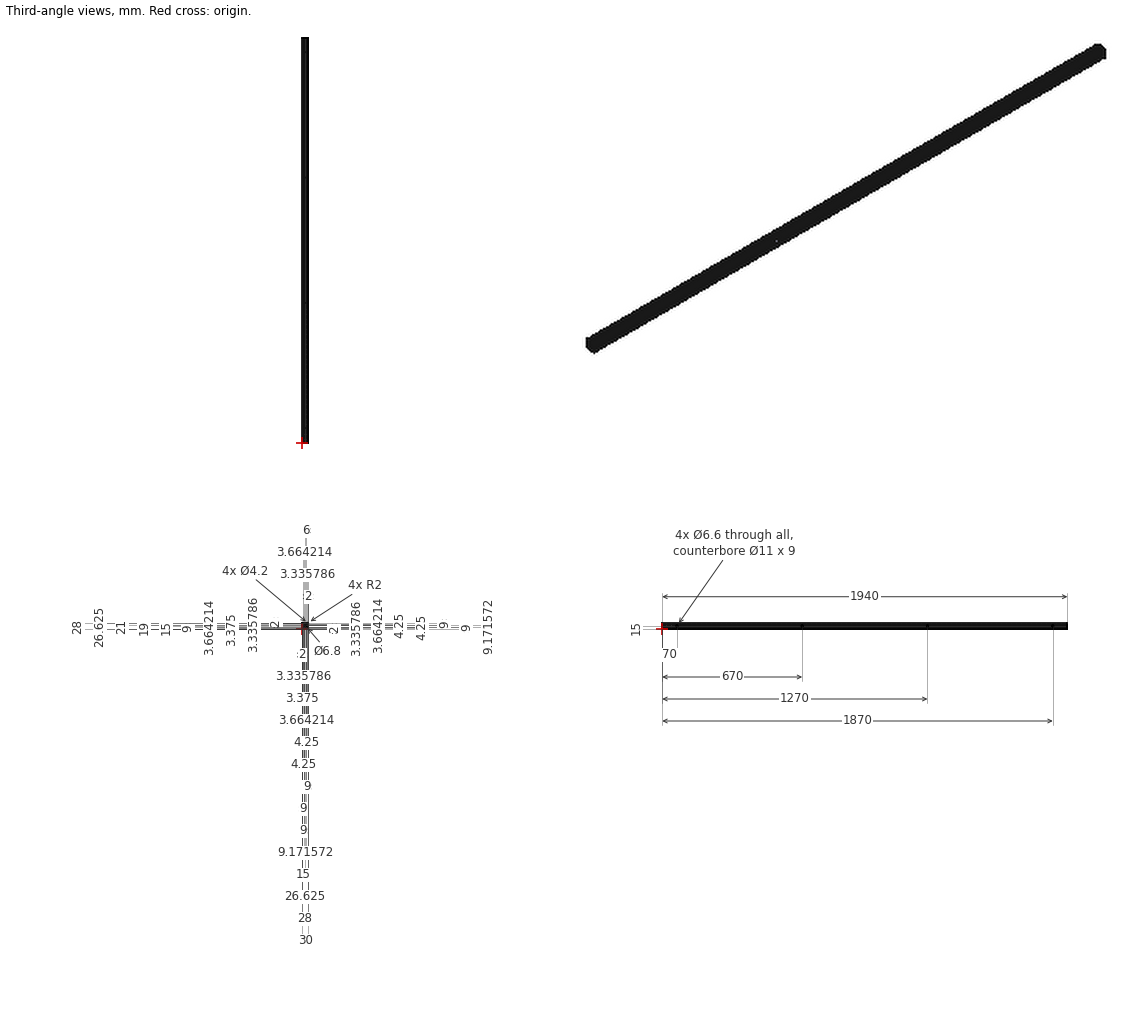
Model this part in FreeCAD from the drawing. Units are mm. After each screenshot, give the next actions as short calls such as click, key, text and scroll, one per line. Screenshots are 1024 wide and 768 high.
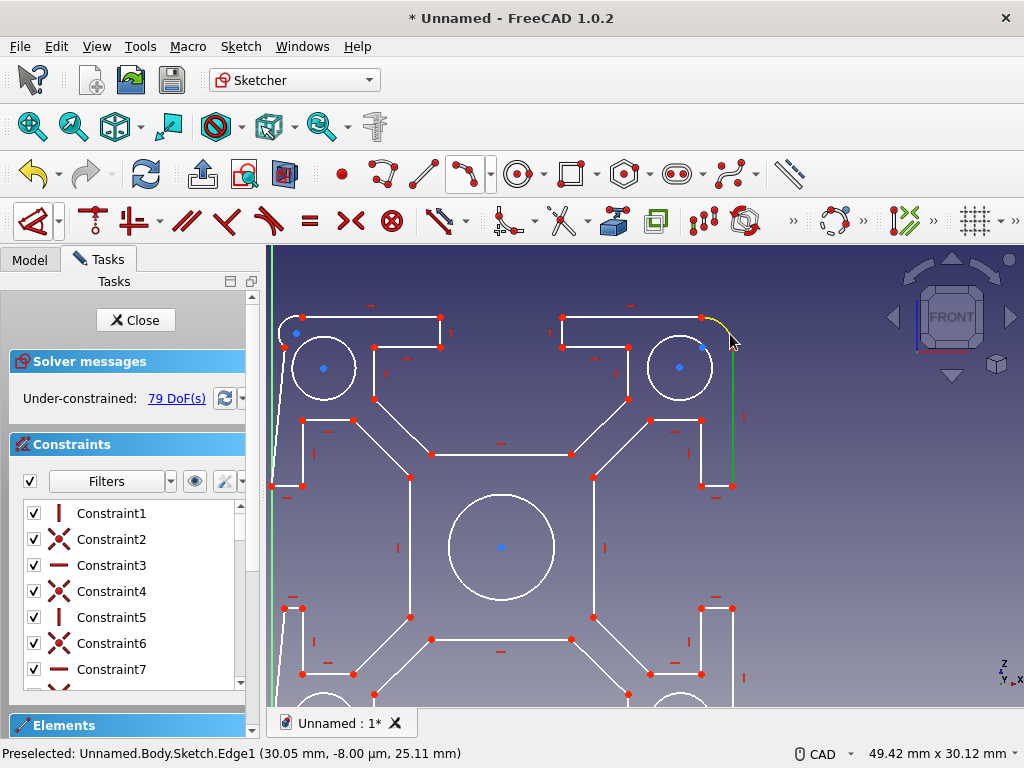
click(729, 333)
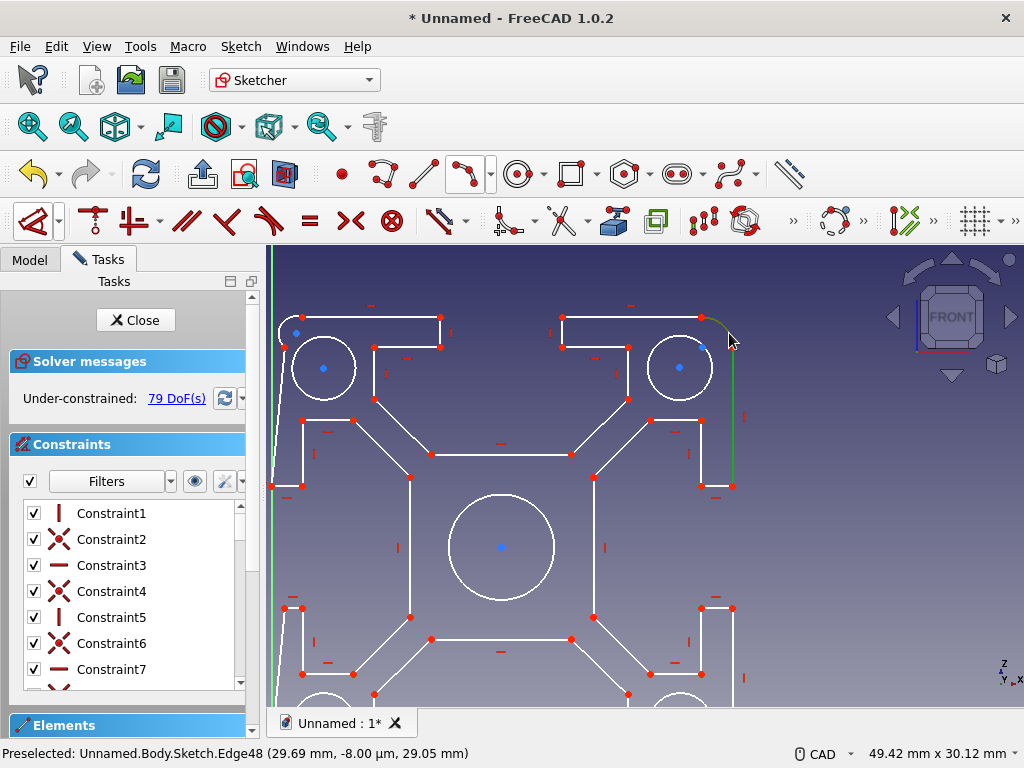
click(269, 222)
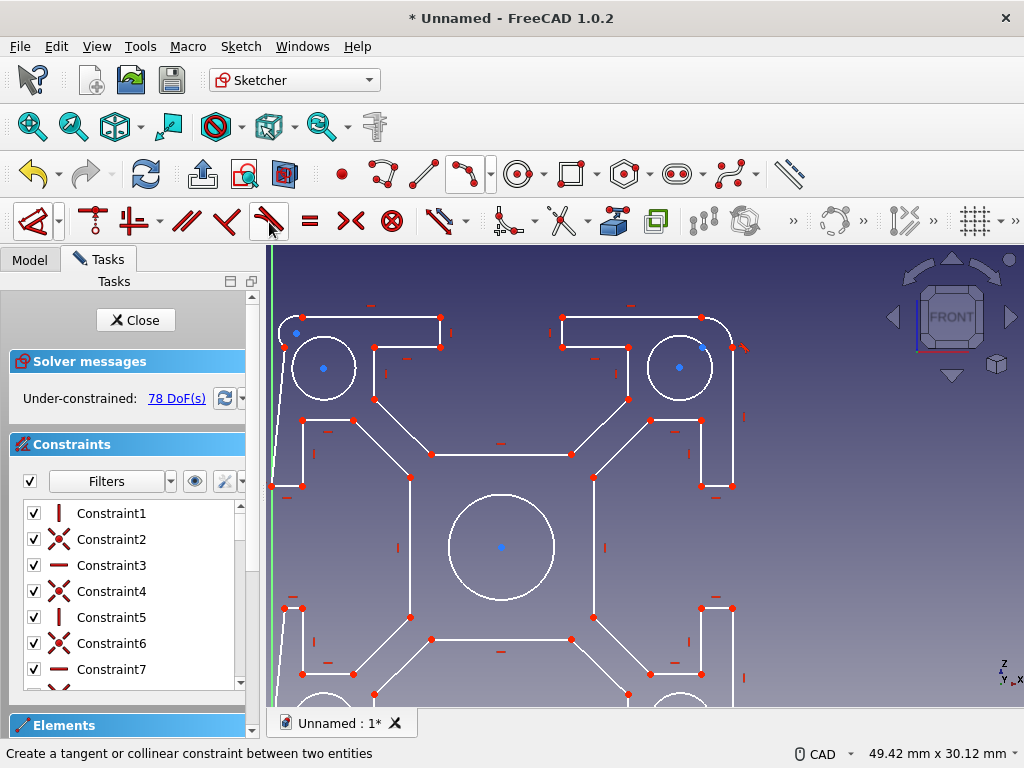
click(733, 650)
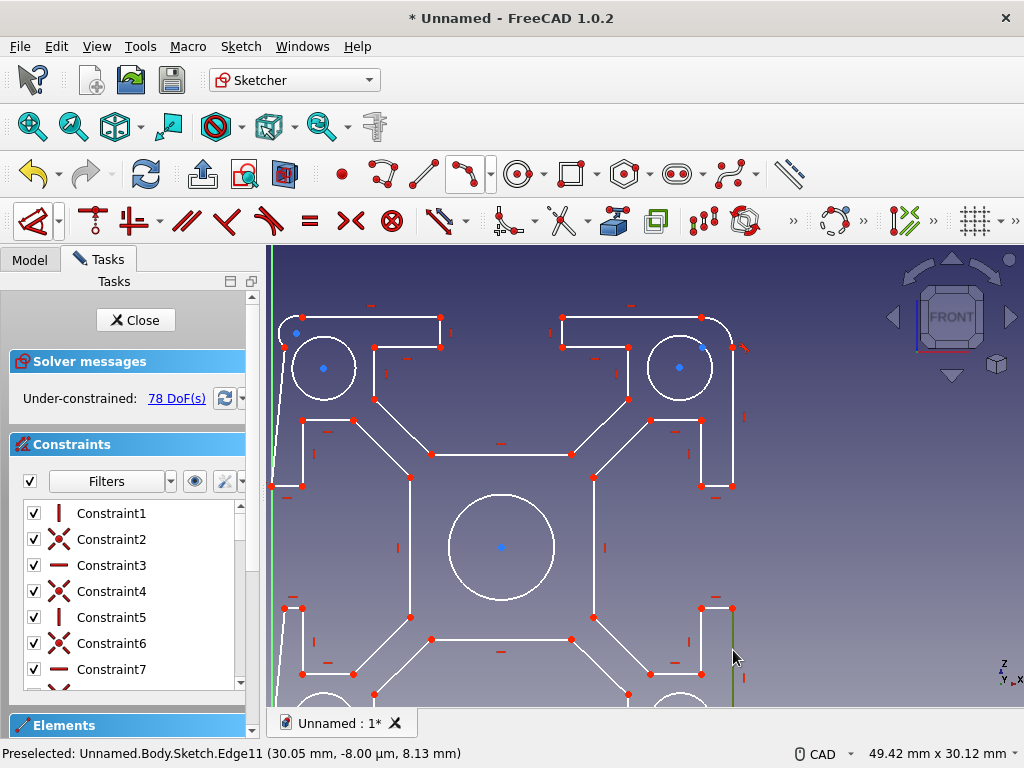
scroll(729, 334, down, 2)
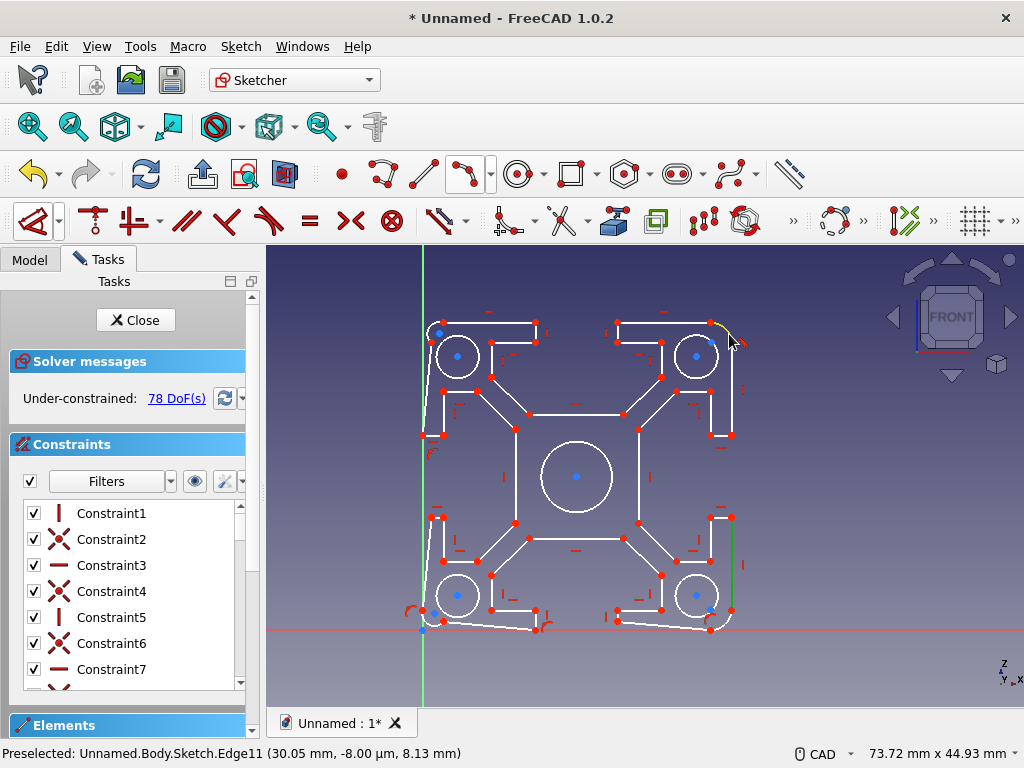
scroll(720, 628, up, 2)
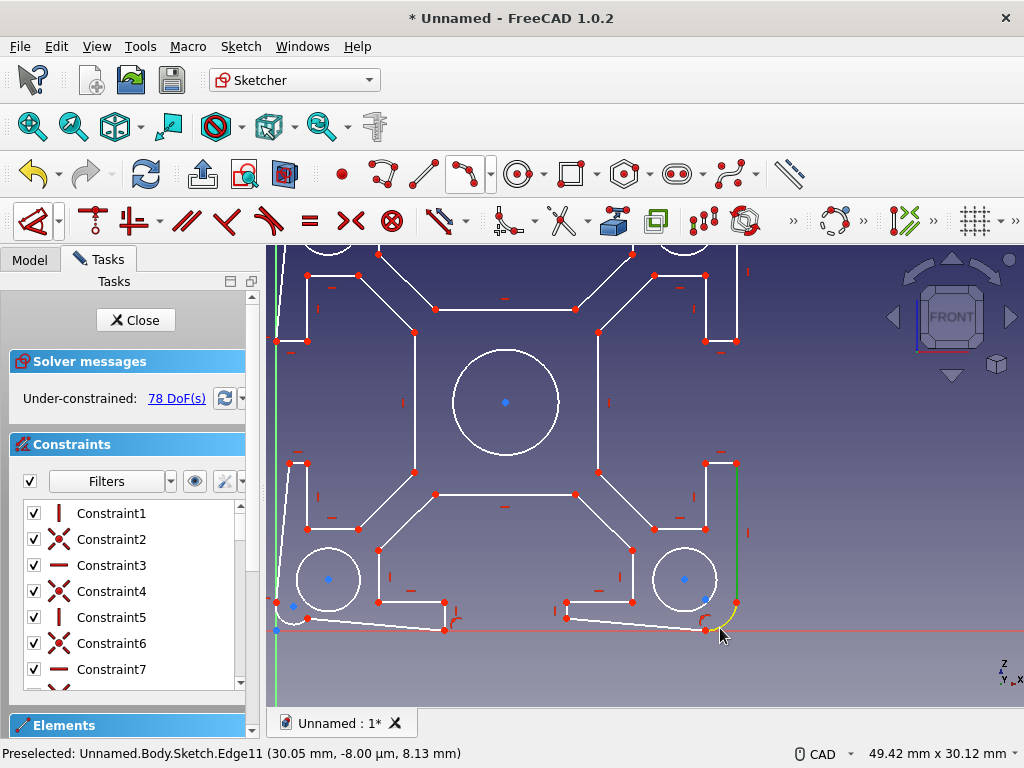
click(719, 628)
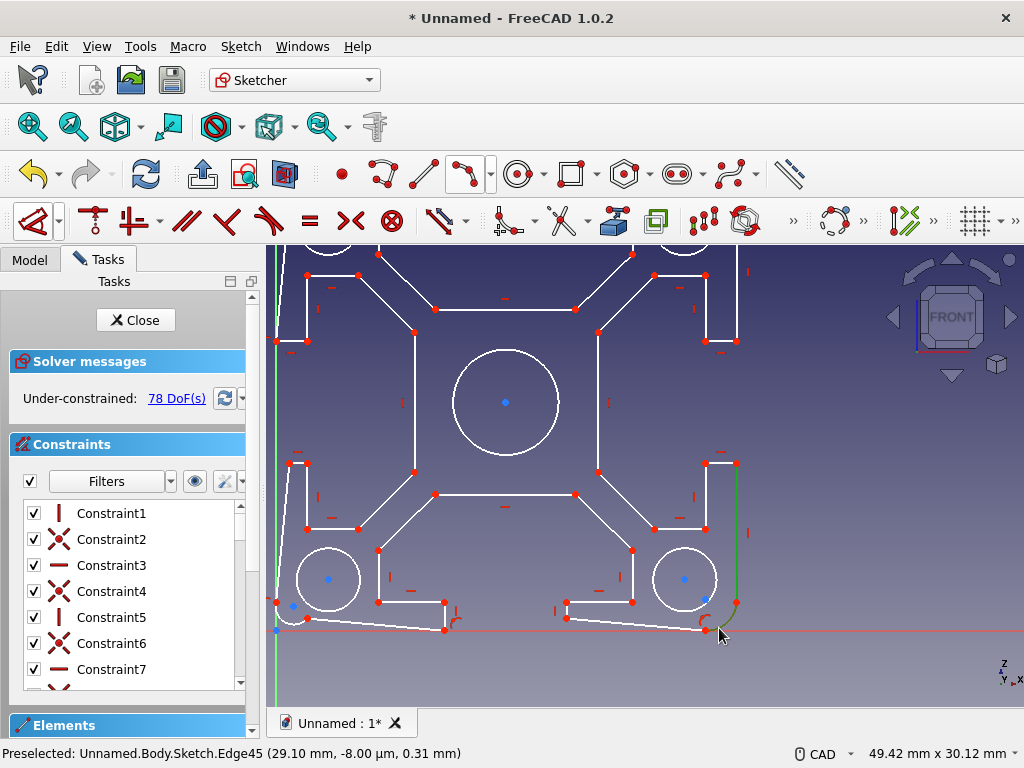
key(t)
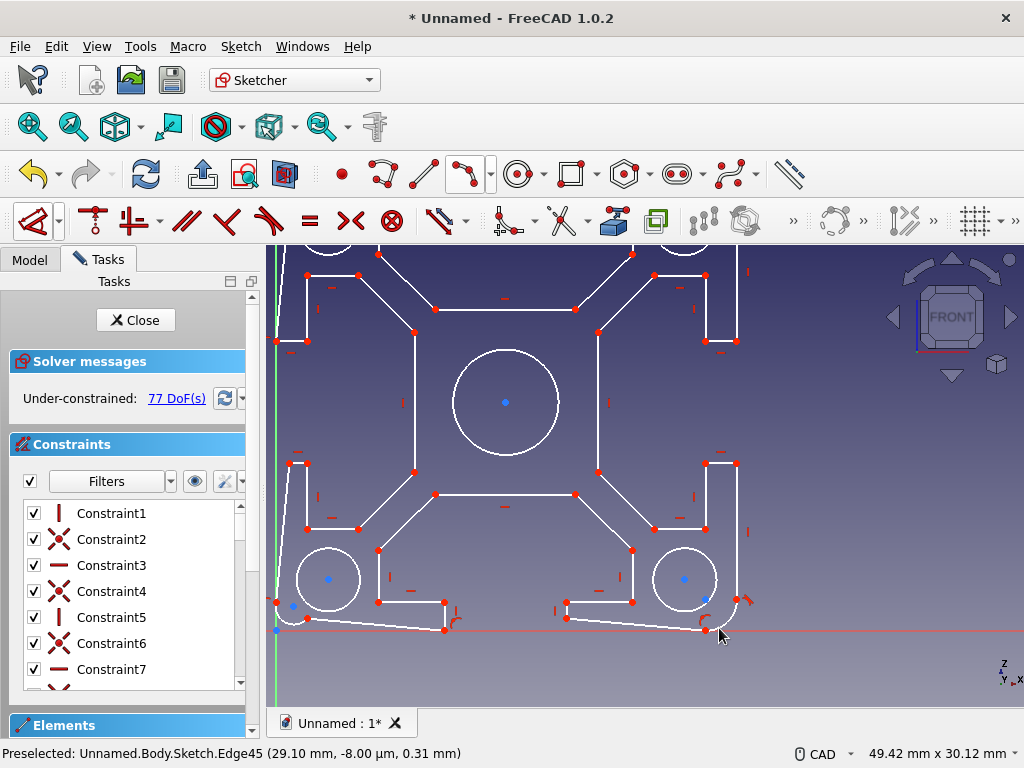
click(664, 627)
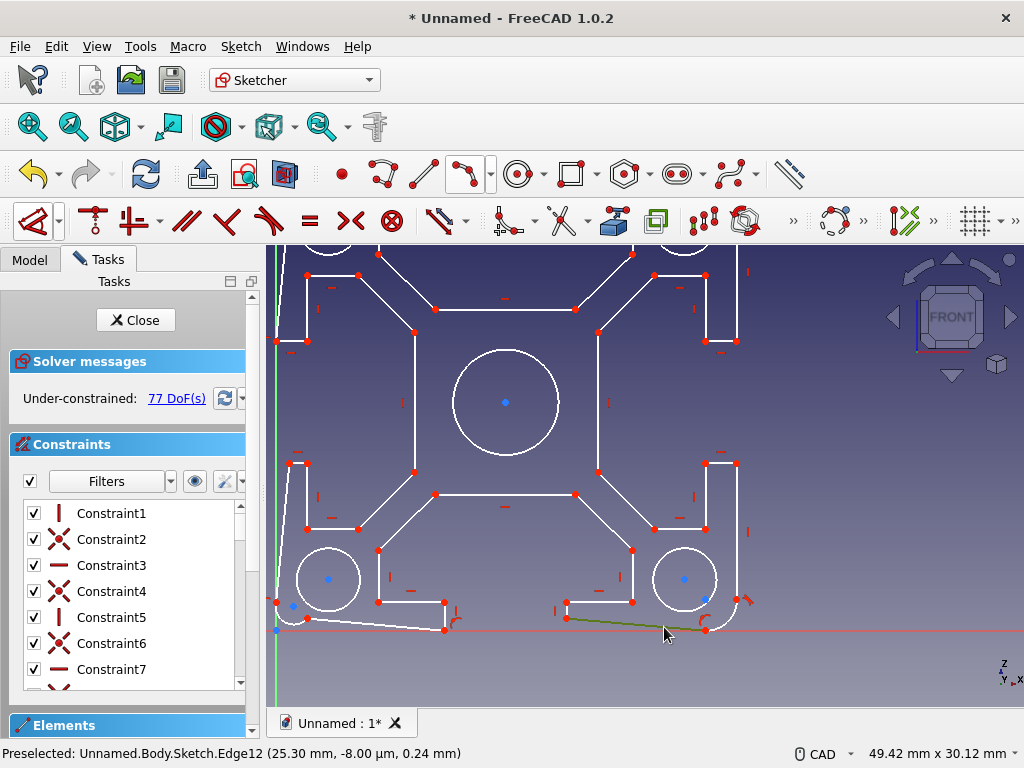
click(720, 627)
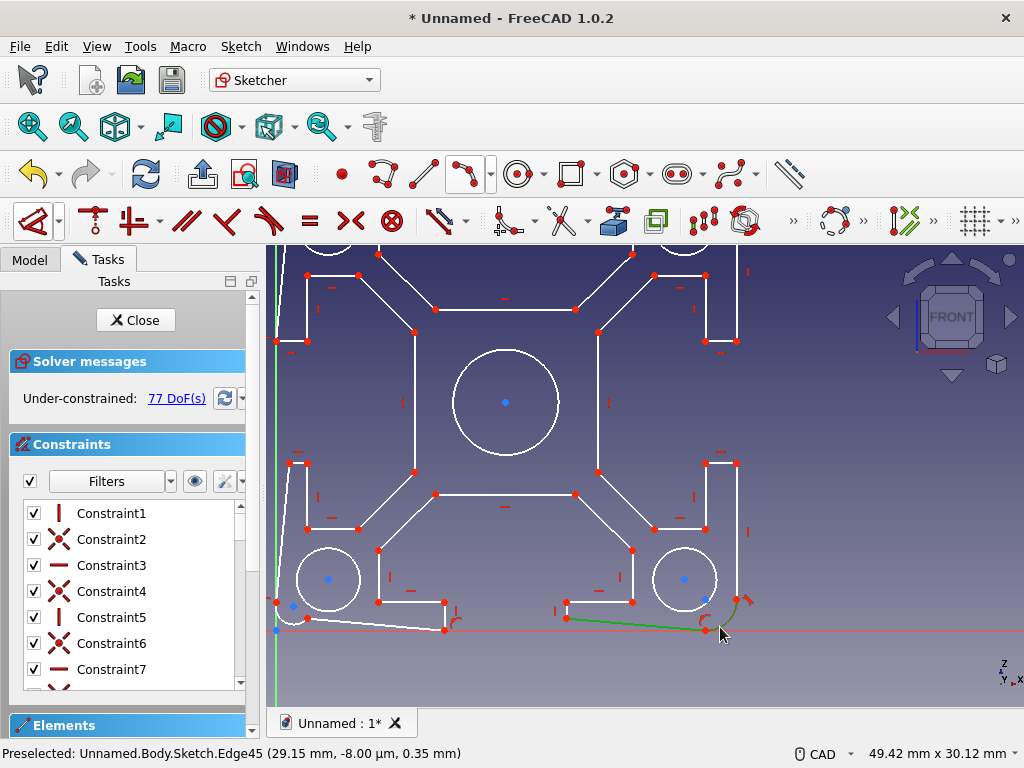
key(t)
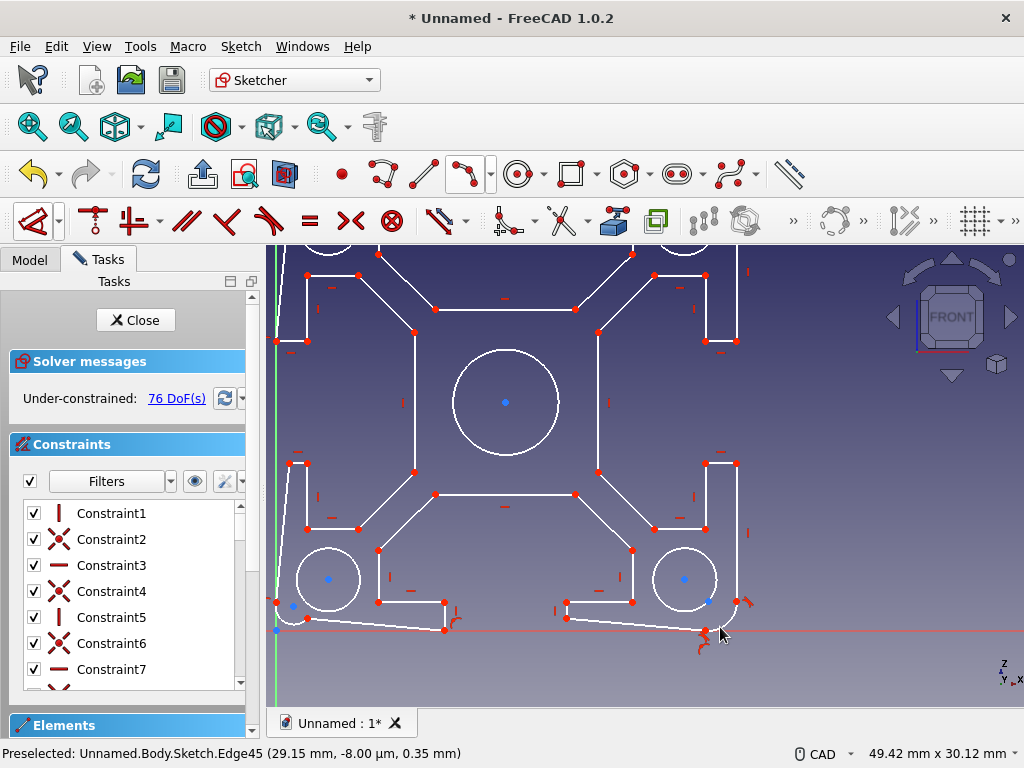
click(403, 627)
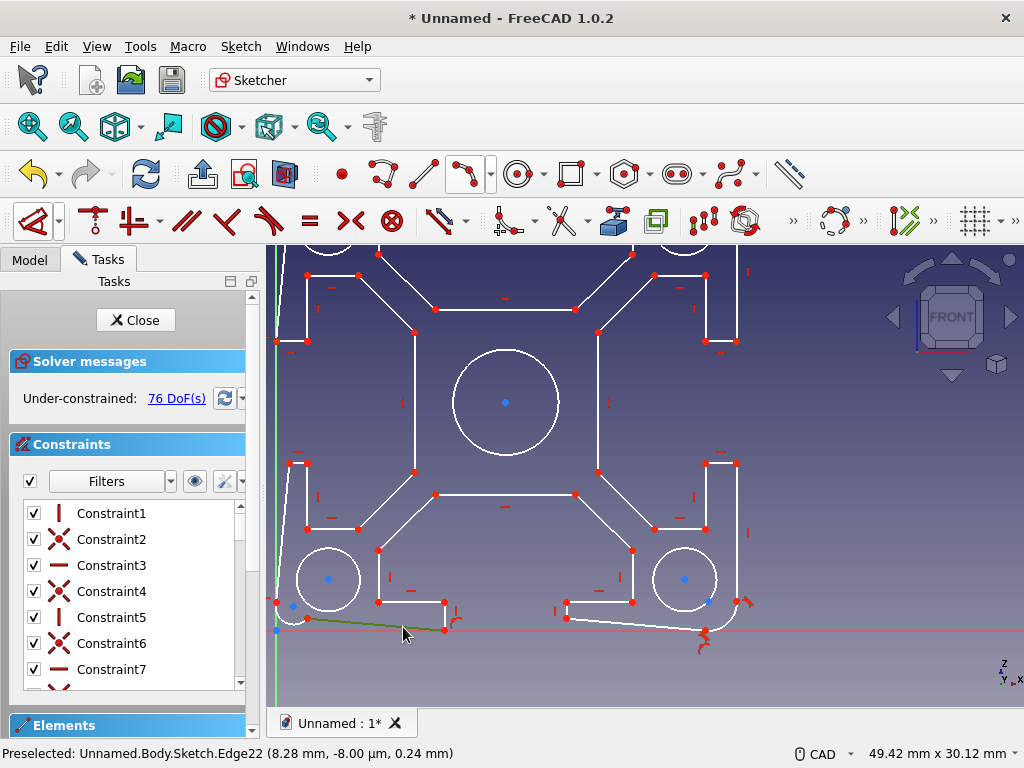
scroll(720, 629, down, 2)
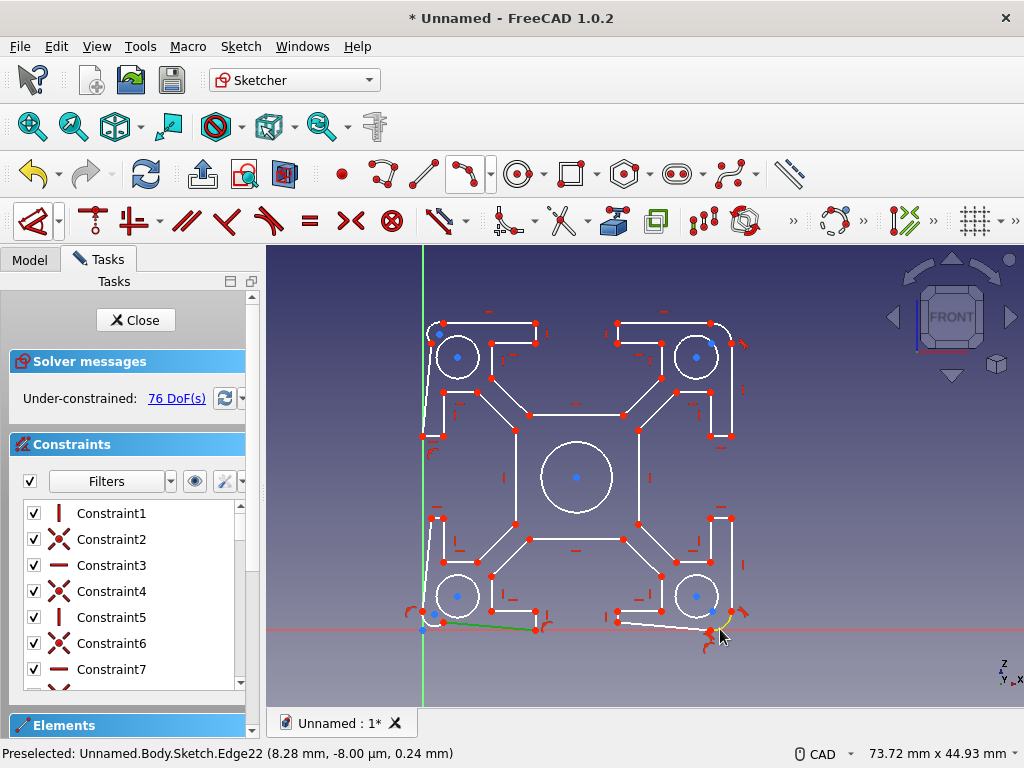
scroll(424, 621, up, 2)